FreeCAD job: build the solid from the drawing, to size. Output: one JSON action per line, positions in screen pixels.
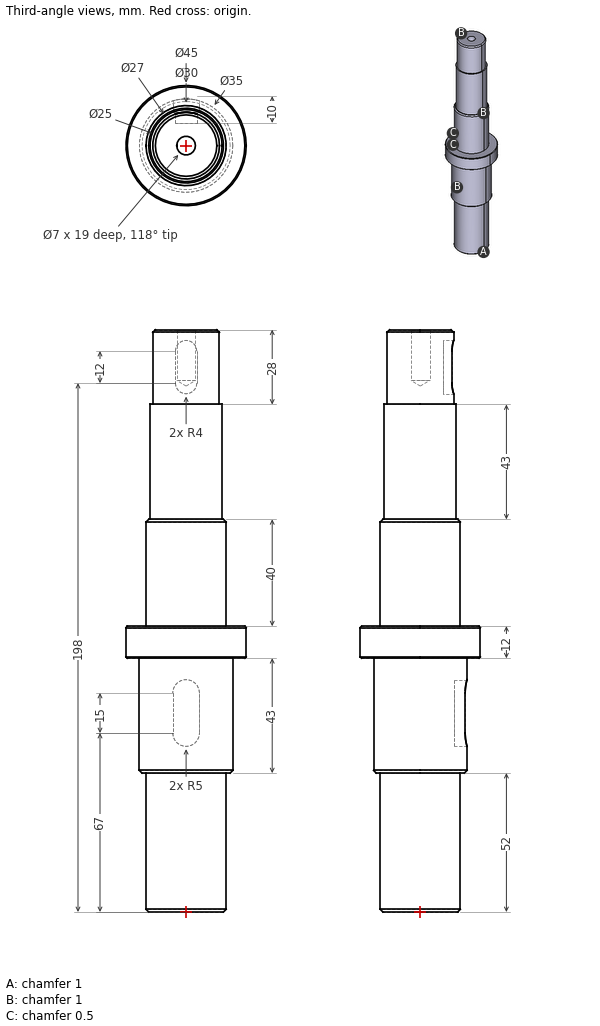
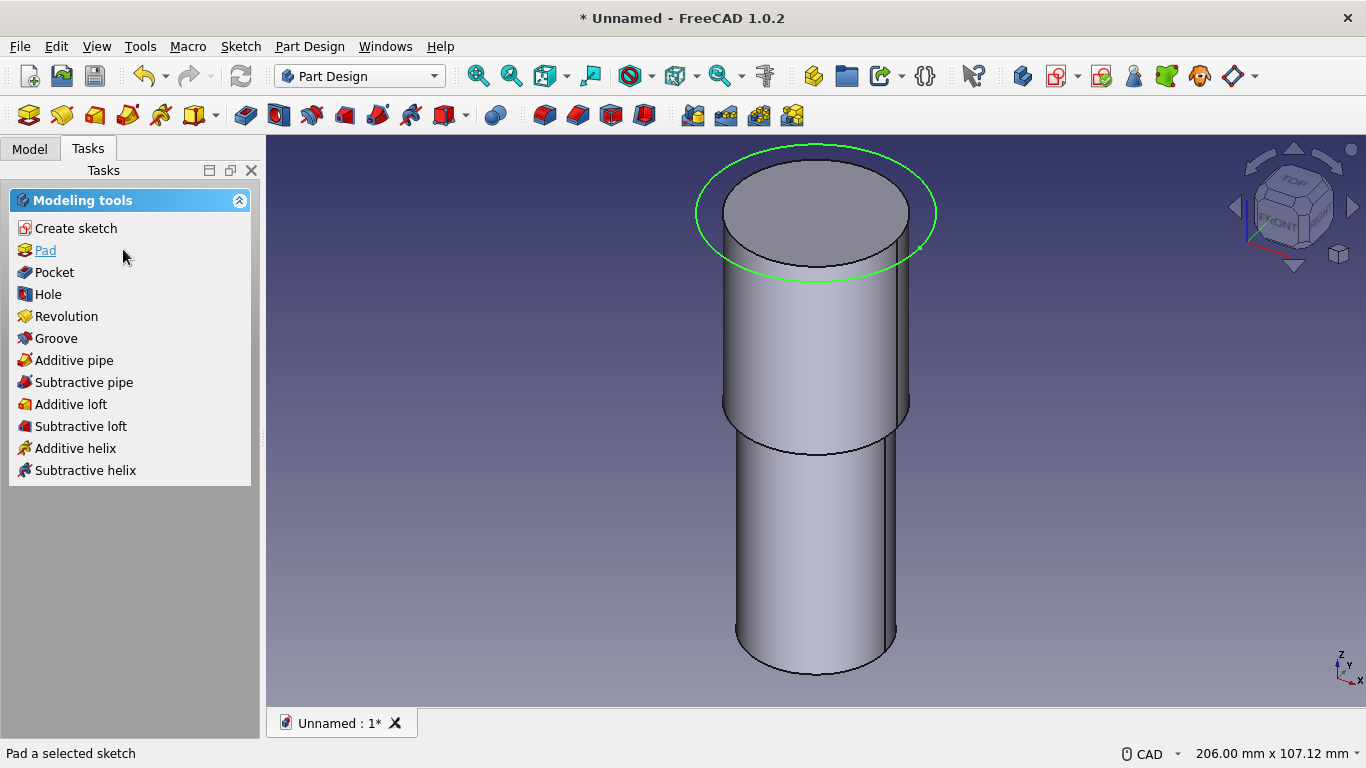
{"action": "left_click", "coordinate": [29, 116]}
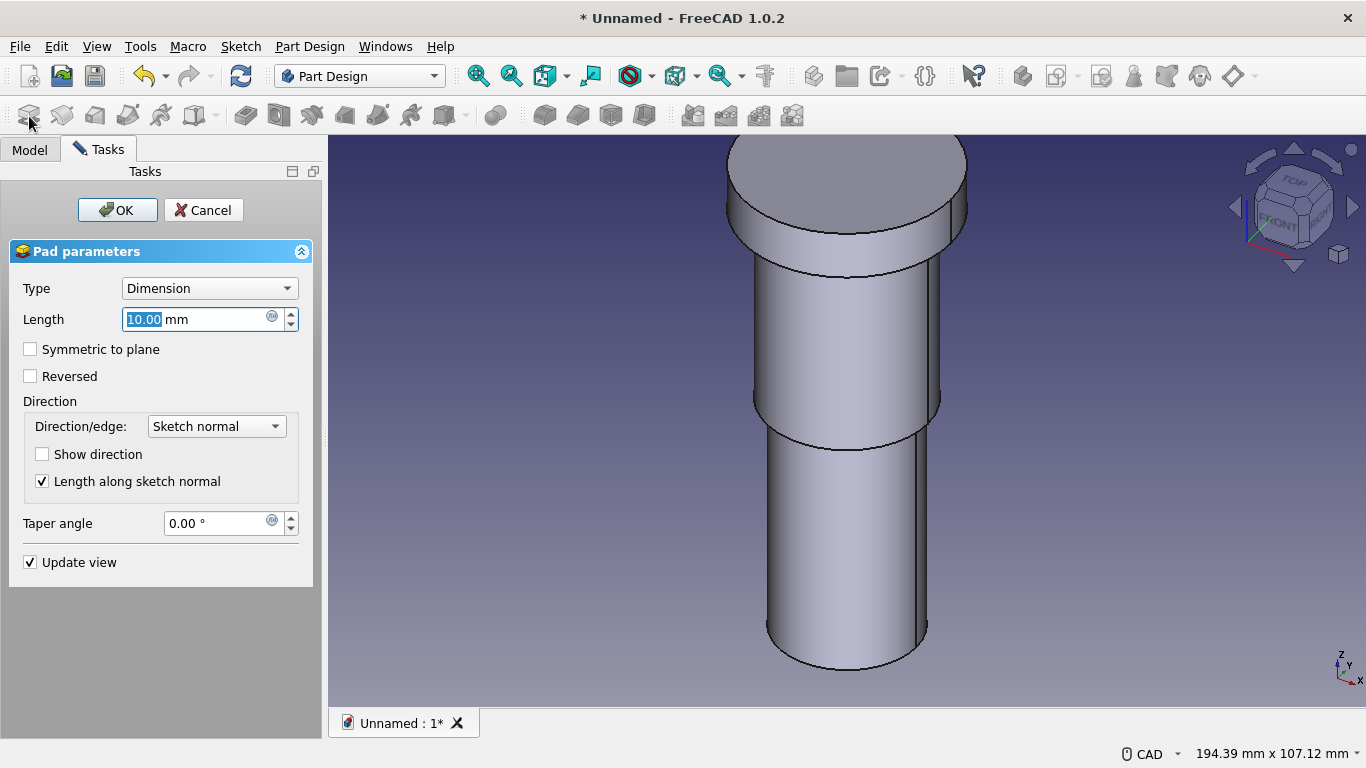
{"action": "type", "text": "12"}
{"action": "key", "text": "Tab"}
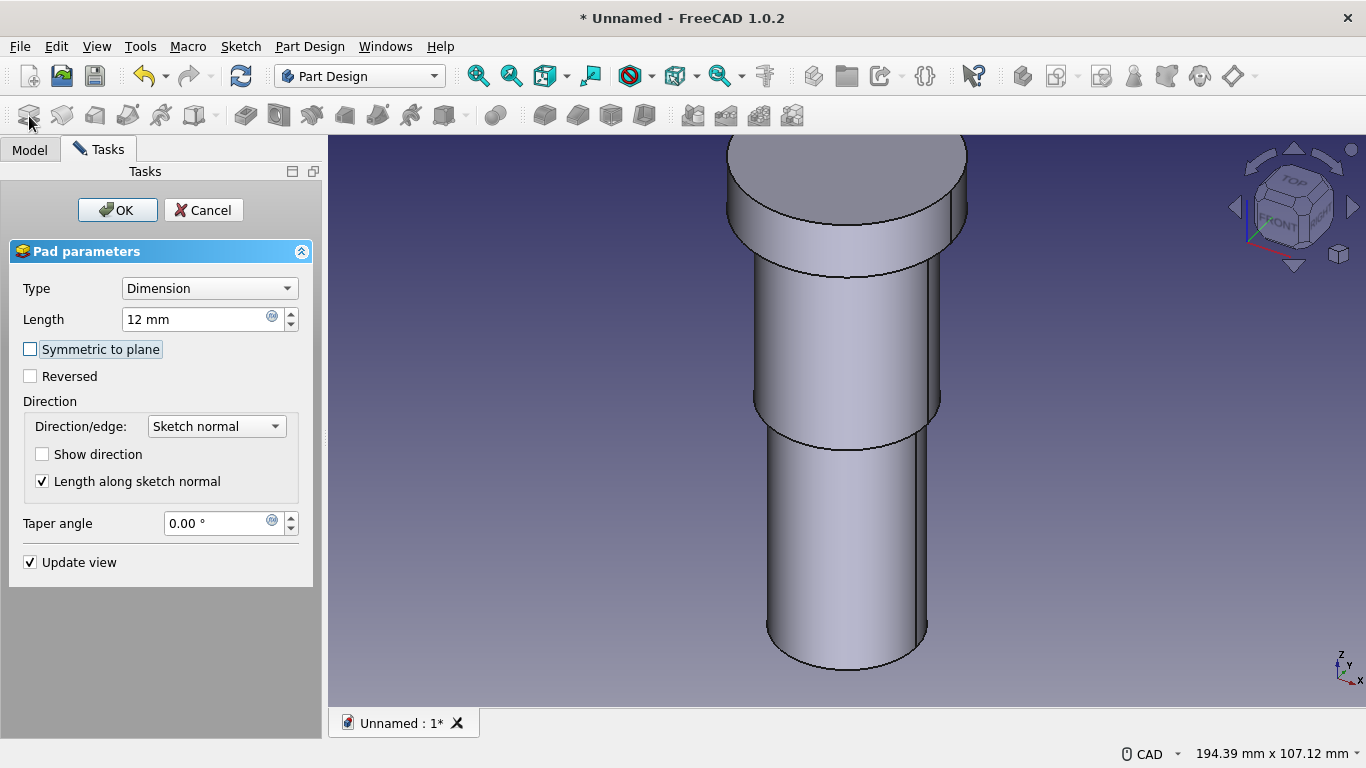
{"action": "left_click", "coordinate": [118, 210]}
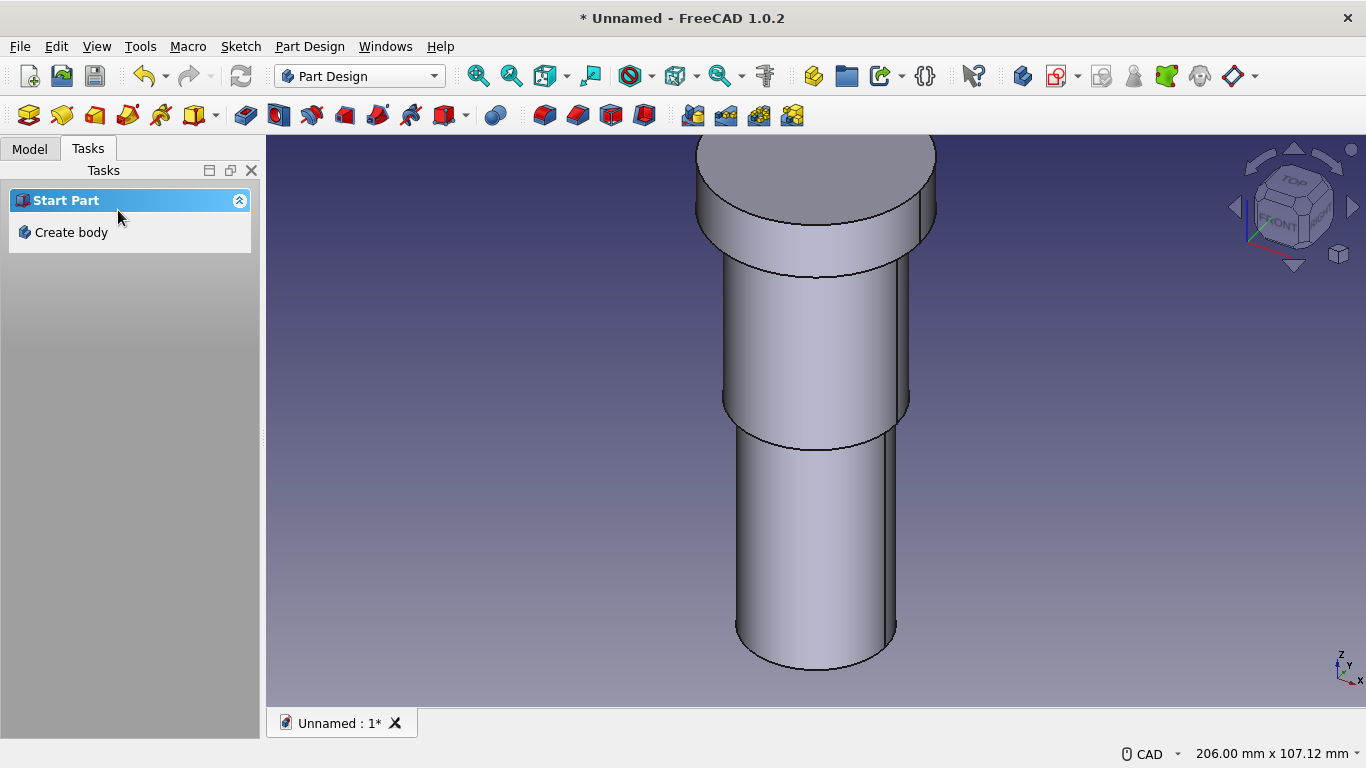
{"action": "key", "text": "v f"}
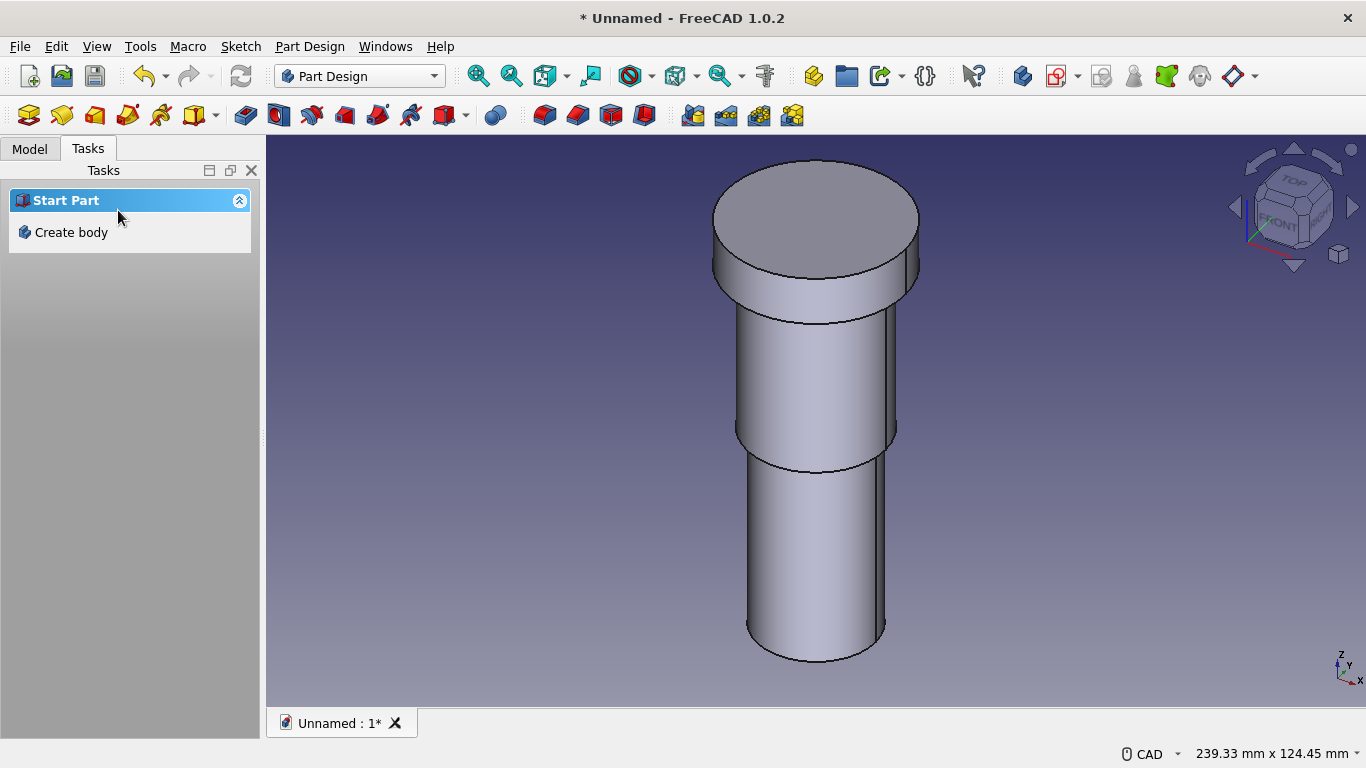
{"action": "left_click", "coordinate": [816, 219]}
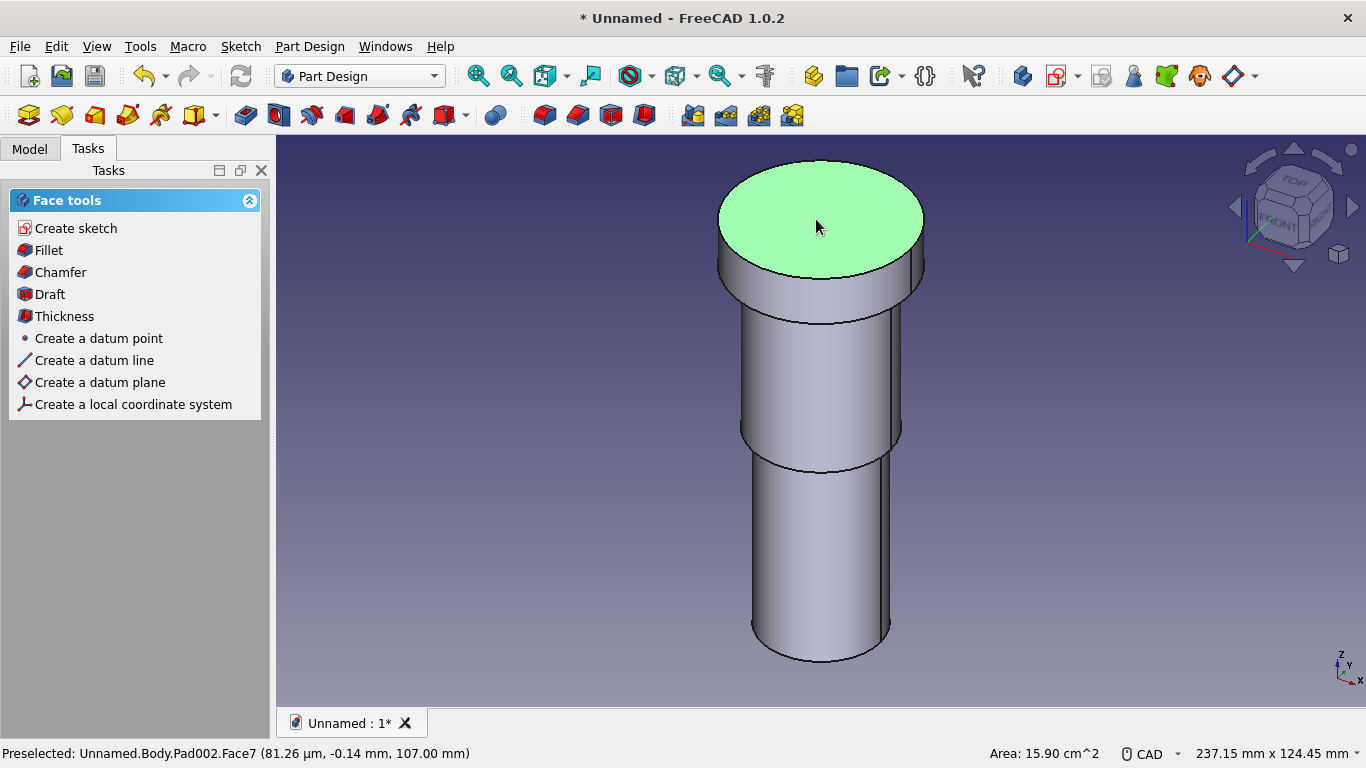
{"action": "left_click", "coordinate": [1056, 76]}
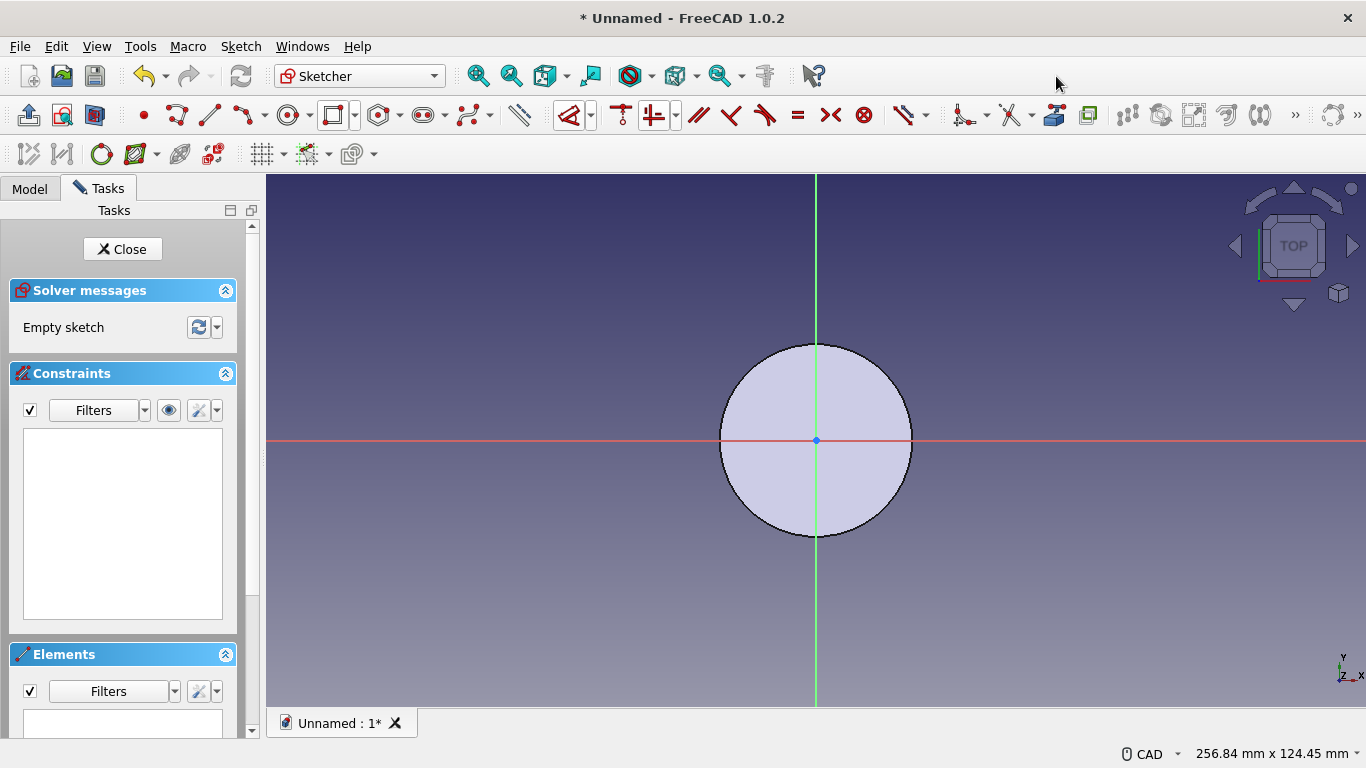
{"action": "scroll", "coordinate": [856, 440], "scroll_direction": "up", "scroll_amount": 5}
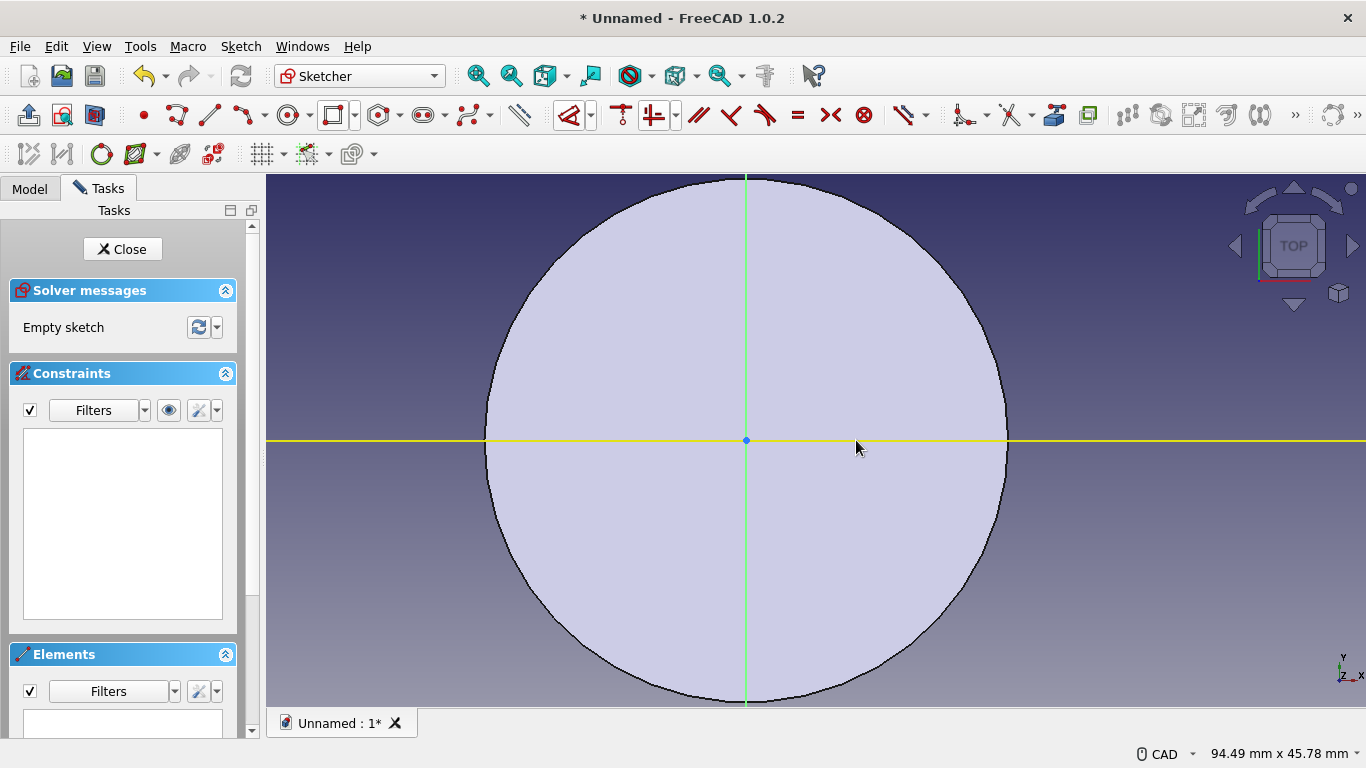
{"action": "left_click", "coordinate": [288, 116]}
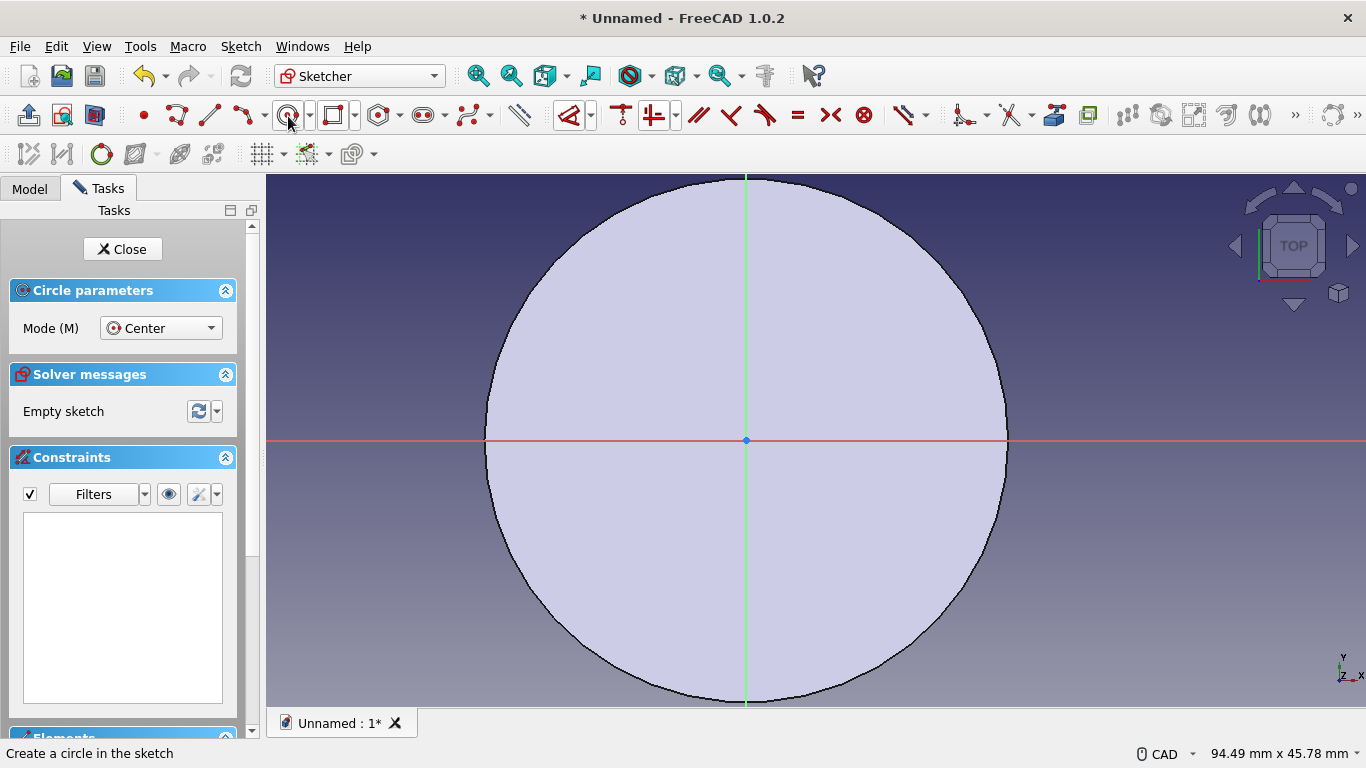
{"action": "left_click", "coordinate": [746, 440]}
{"action": "mouse_move", "coordinate": [870, 317]}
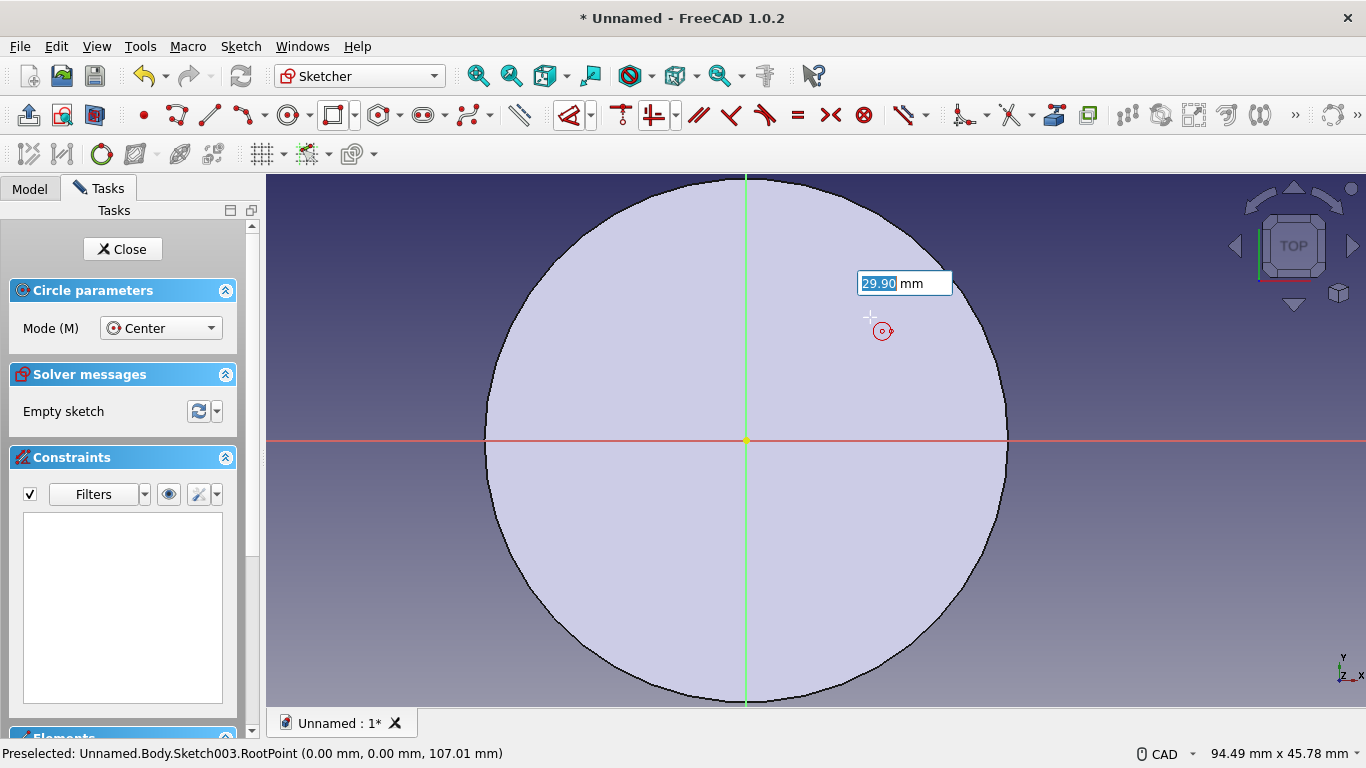
{"action": "type", "text": "30"}
{"action": "key", "text": "Return"}
{"action": "key", "text": "Escape"}